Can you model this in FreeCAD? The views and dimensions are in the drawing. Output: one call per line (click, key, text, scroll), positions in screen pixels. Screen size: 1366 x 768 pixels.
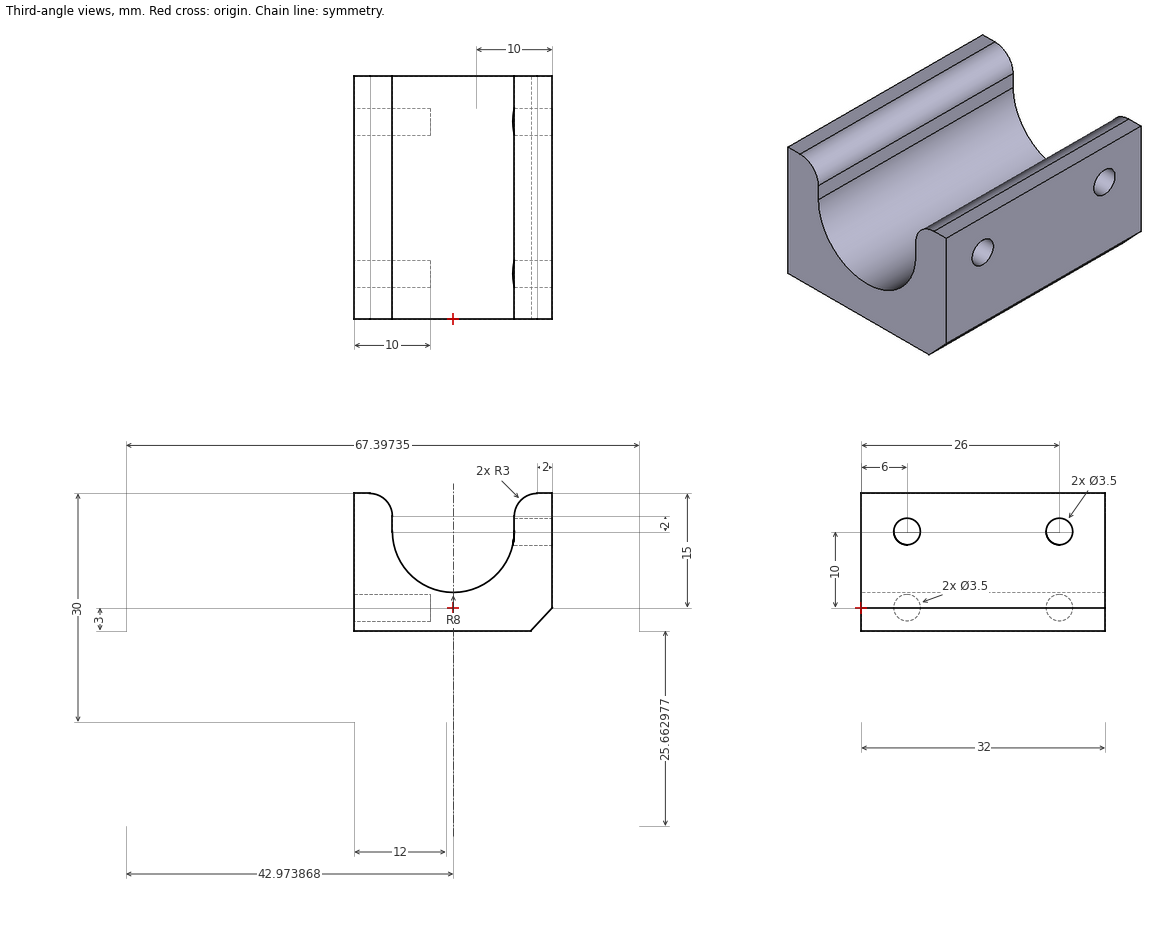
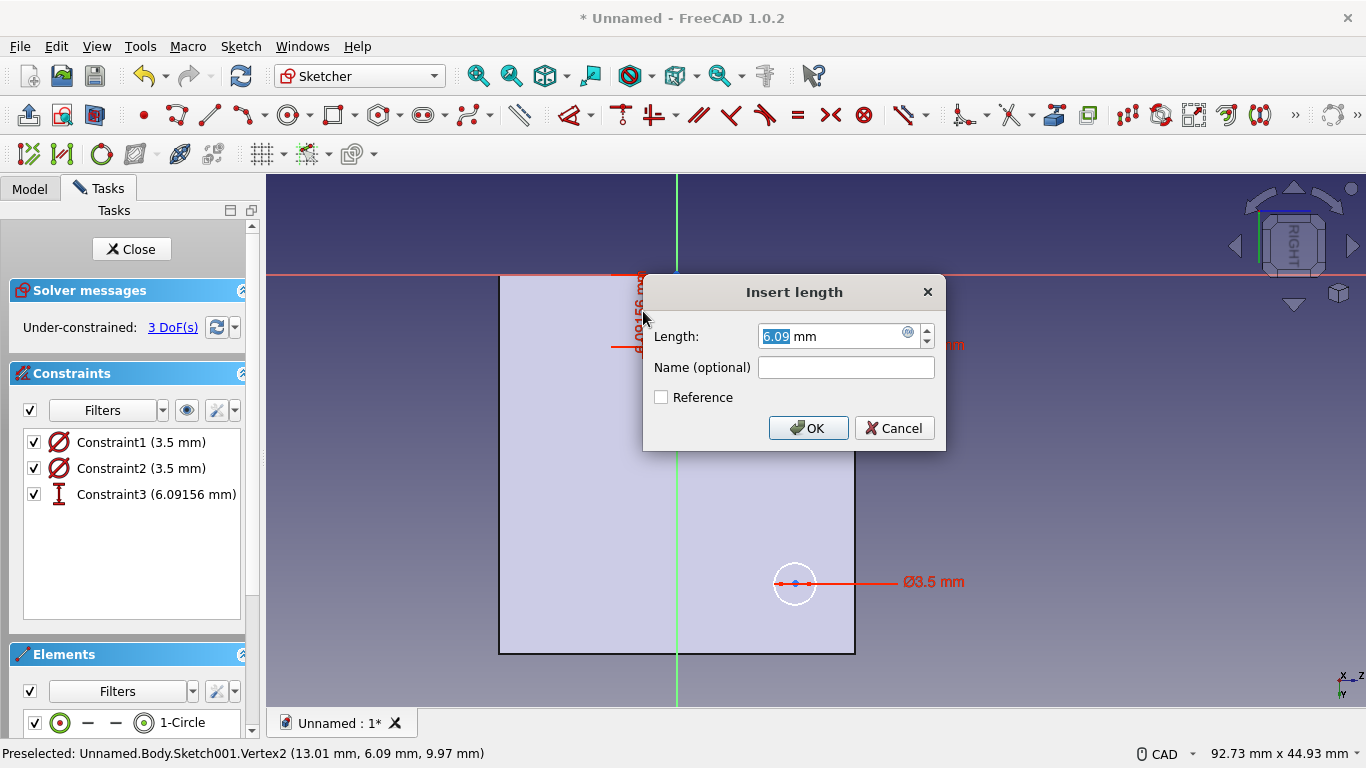
text(6)
key(Return)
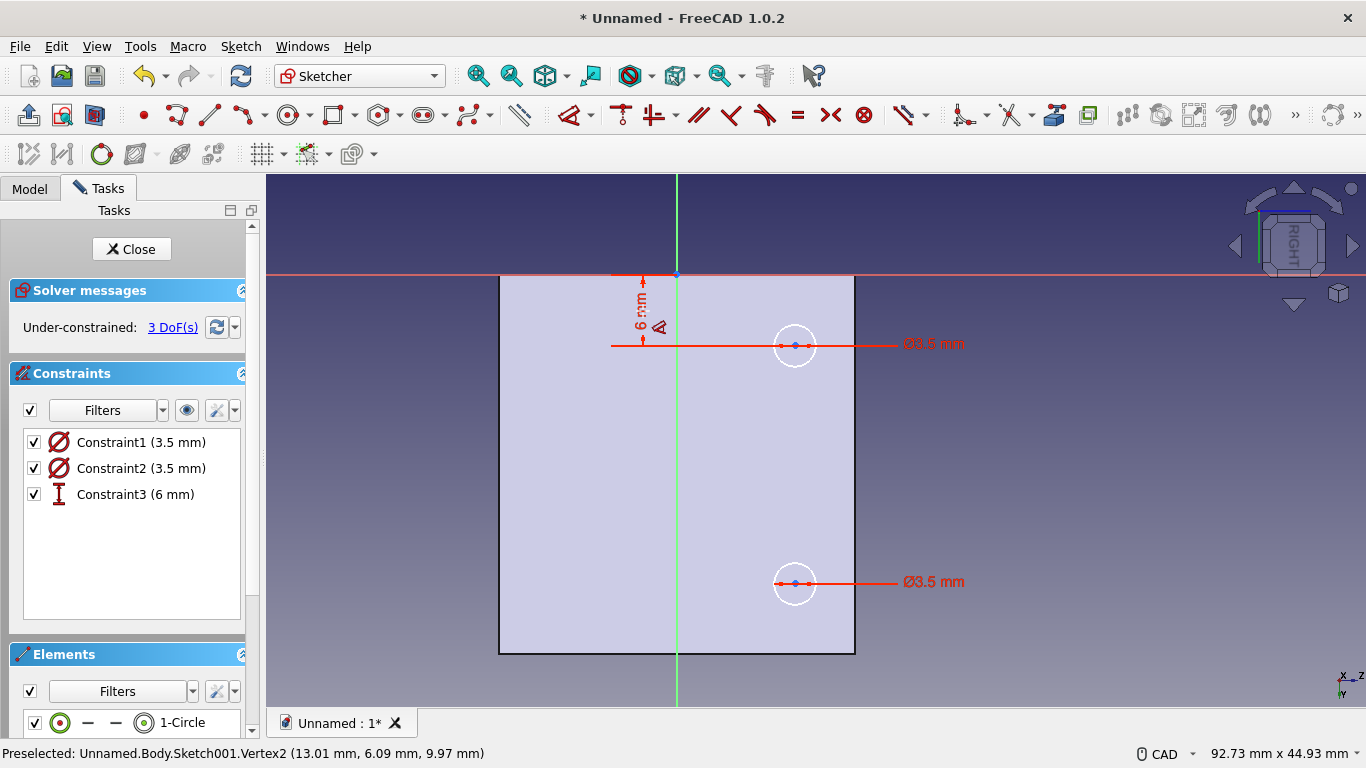
click(795, 584)
click(736, 241)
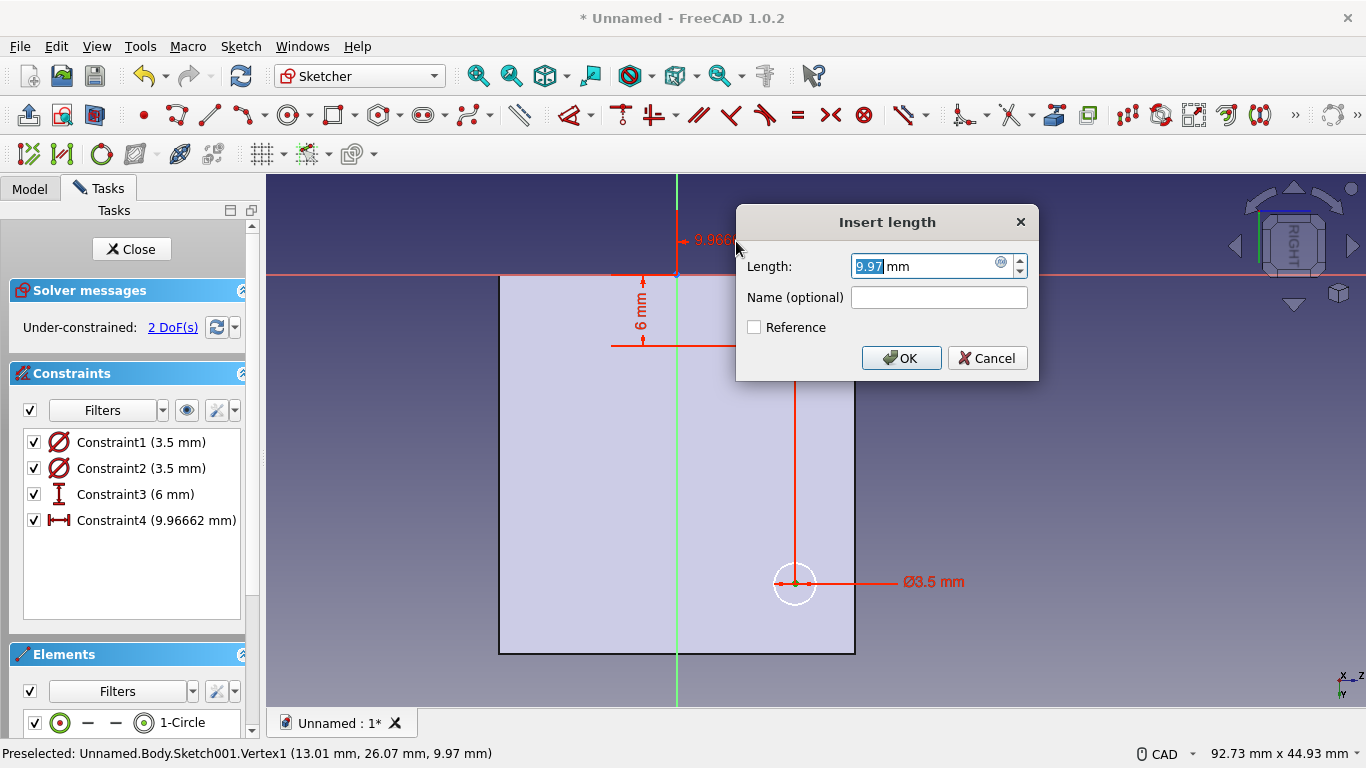
text(10)
key(Return)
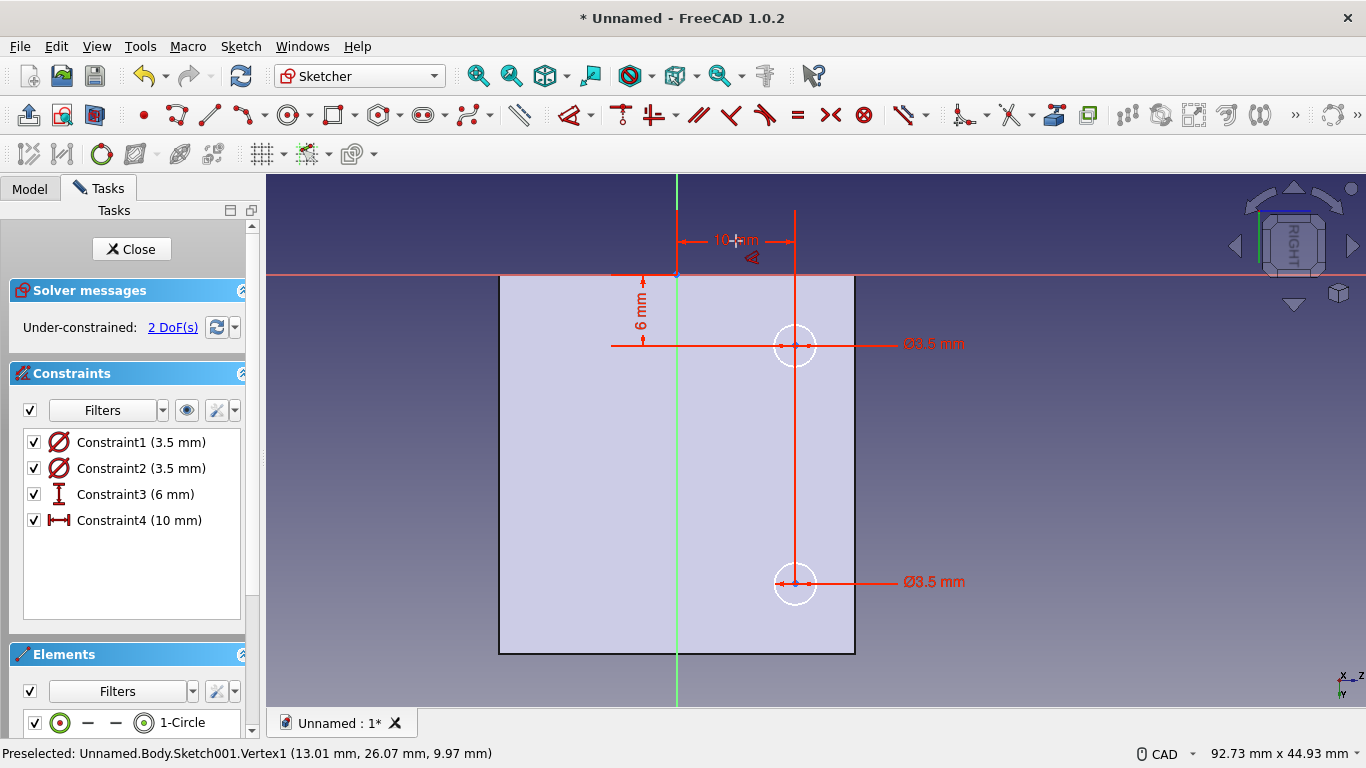
click(795, 584)
click(643, 429)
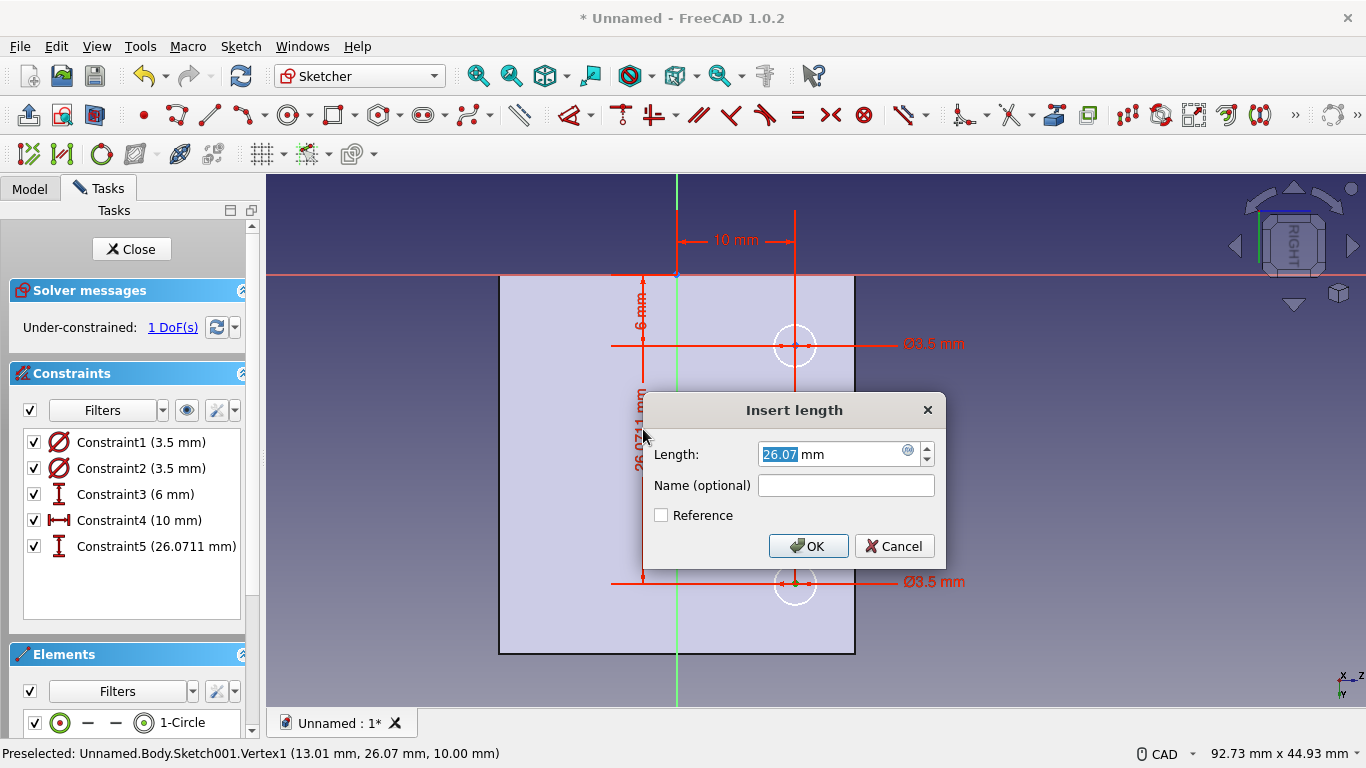
text(26)
key(Return)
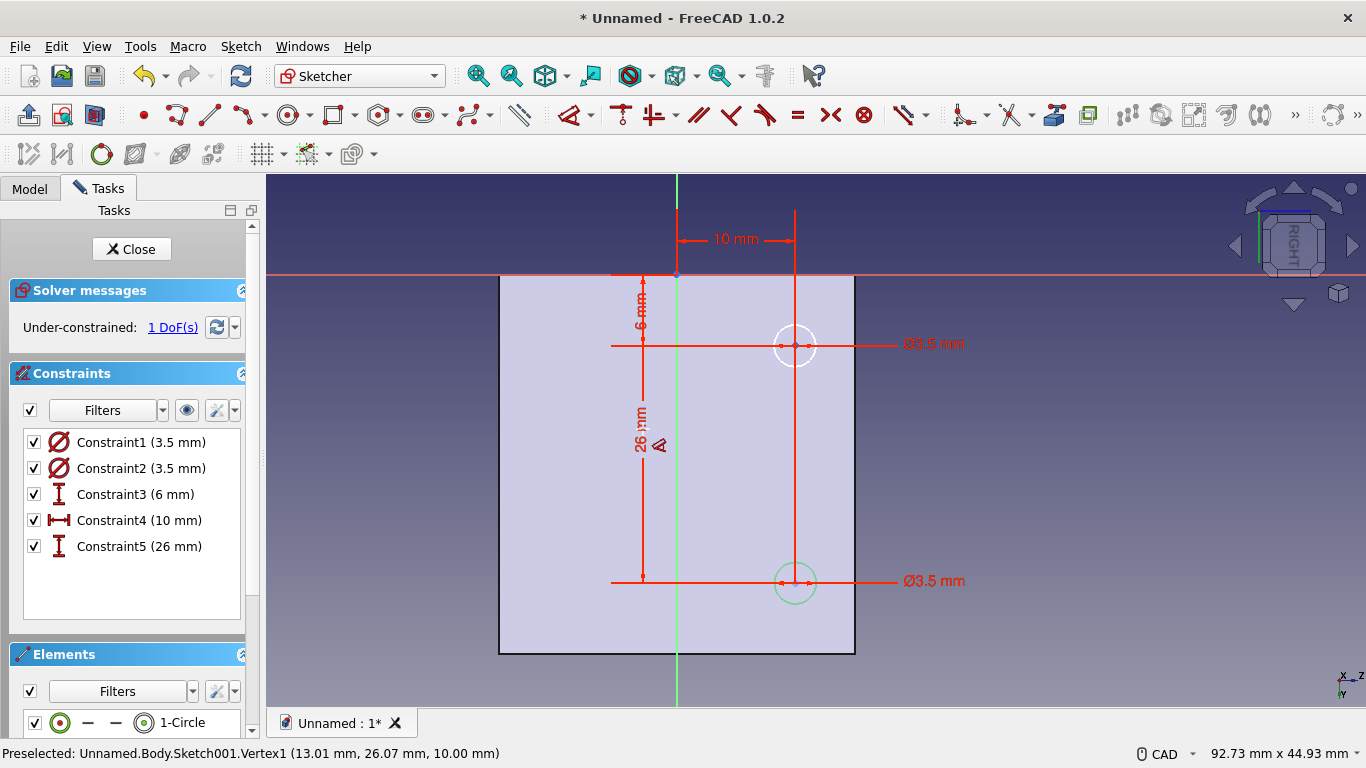
click(795, 346)
click(736, 380)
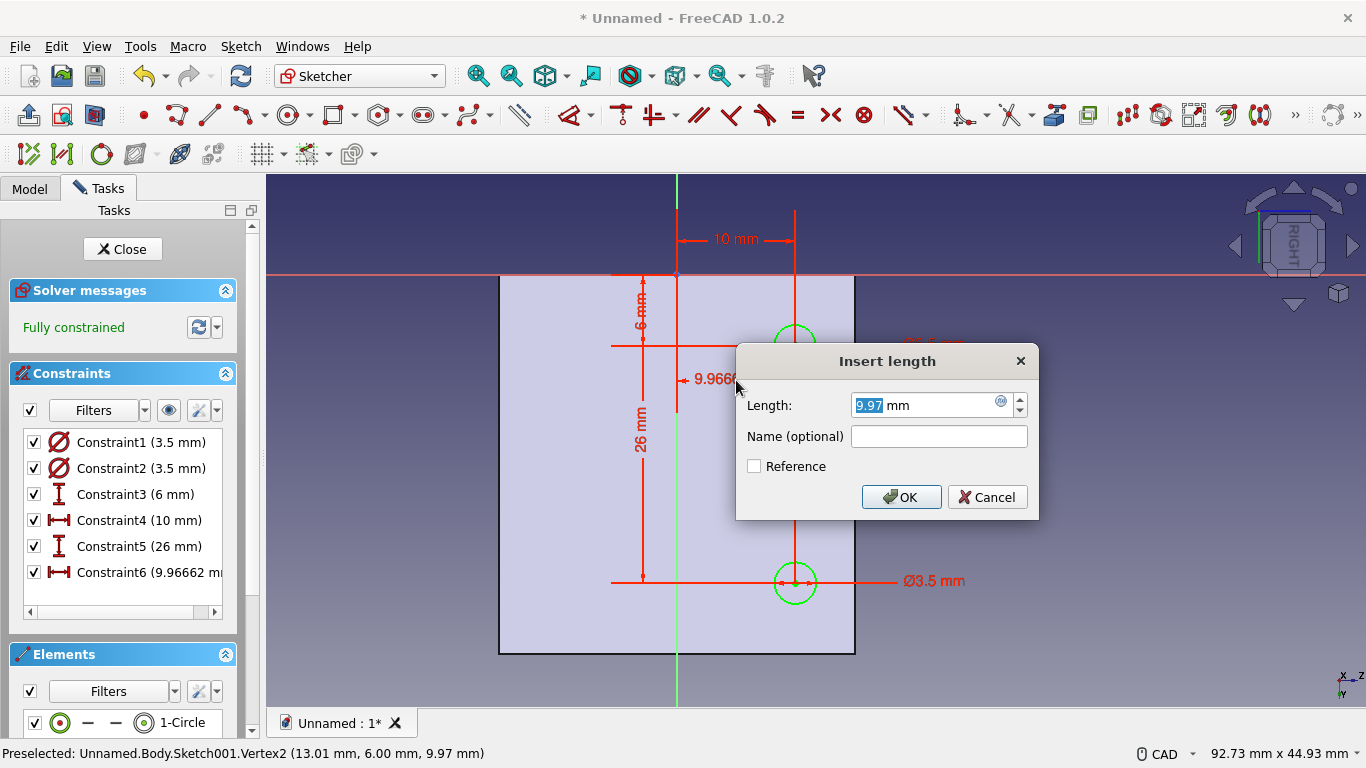
text(10)
key(Return)
key(Escape)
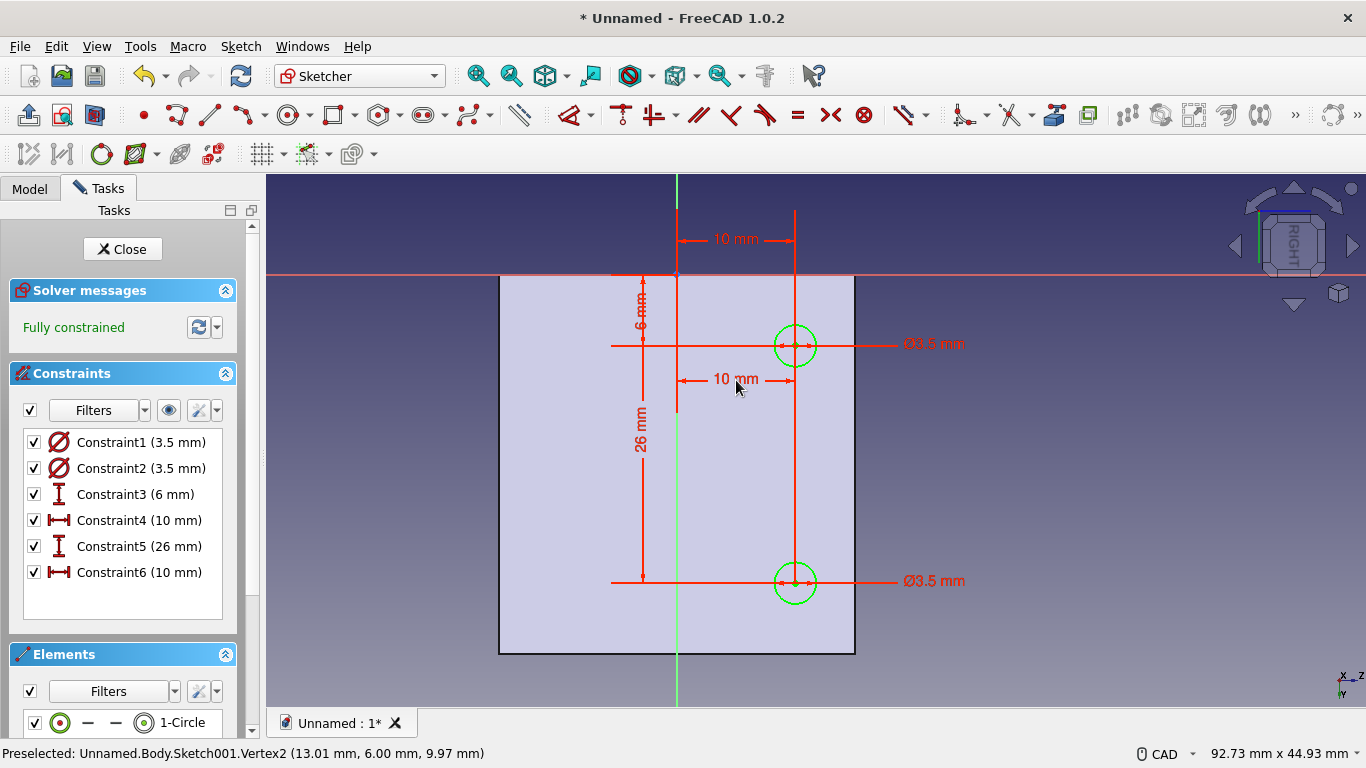
click(123, 249)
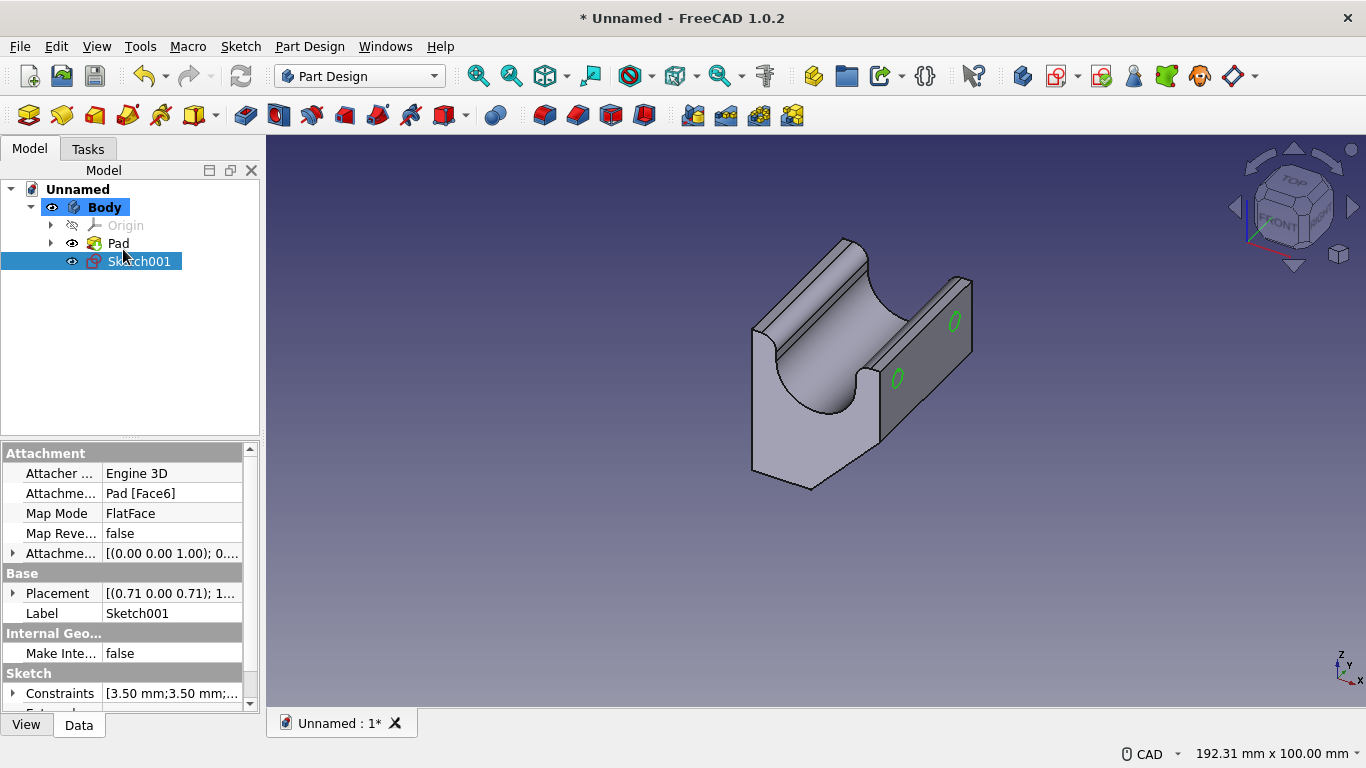
click(246, 116)